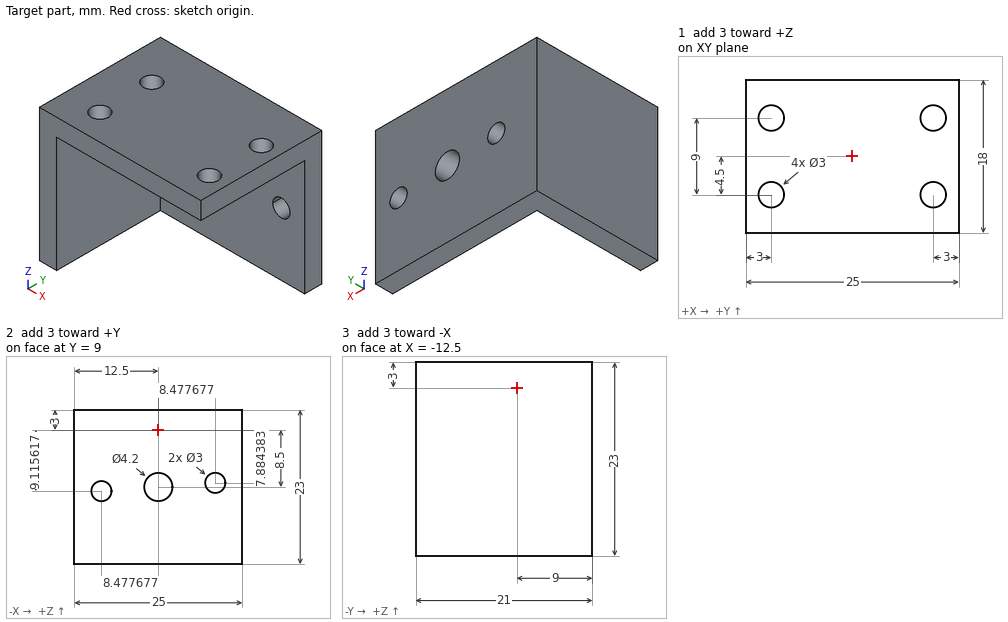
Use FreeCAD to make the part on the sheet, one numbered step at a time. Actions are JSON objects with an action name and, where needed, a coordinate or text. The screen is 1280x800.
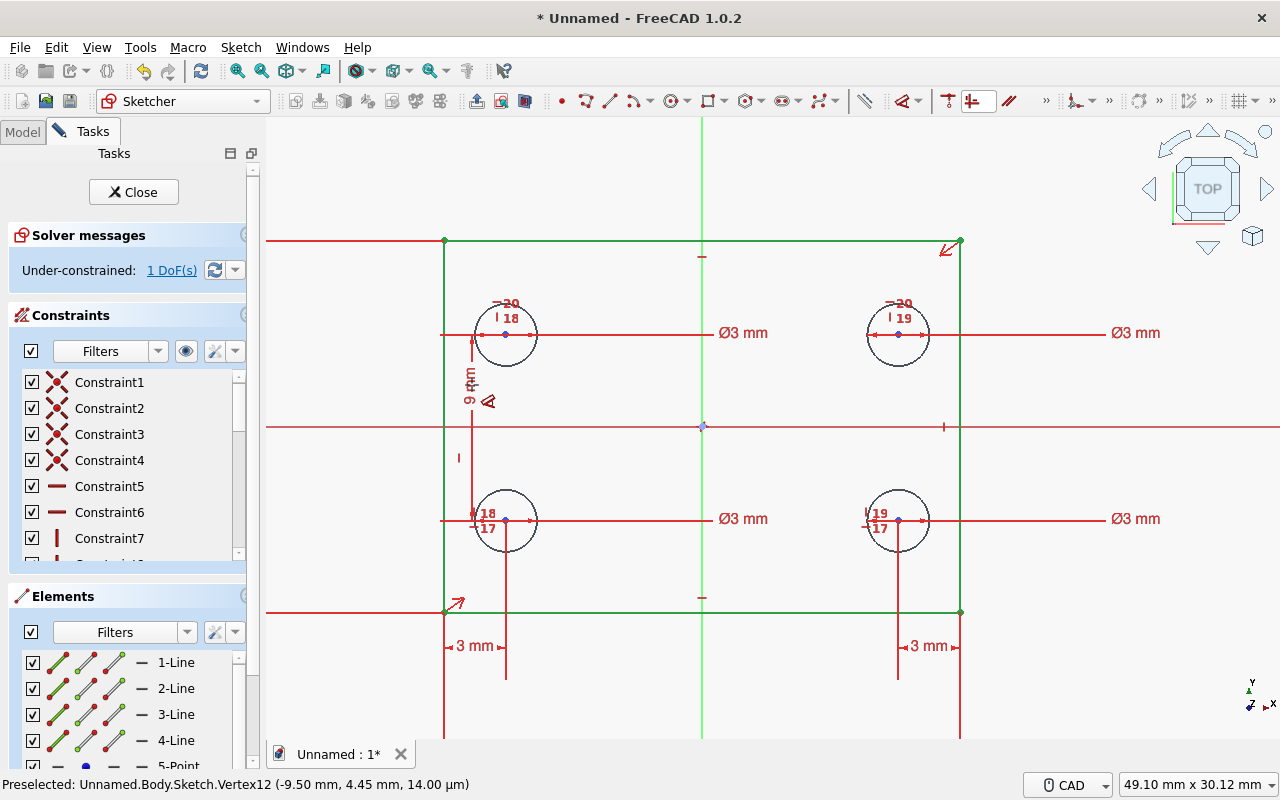
{"action": "left_click", "coordinate": [506, 521]}
{"action": "left_click", "coordinate": [472, 474]}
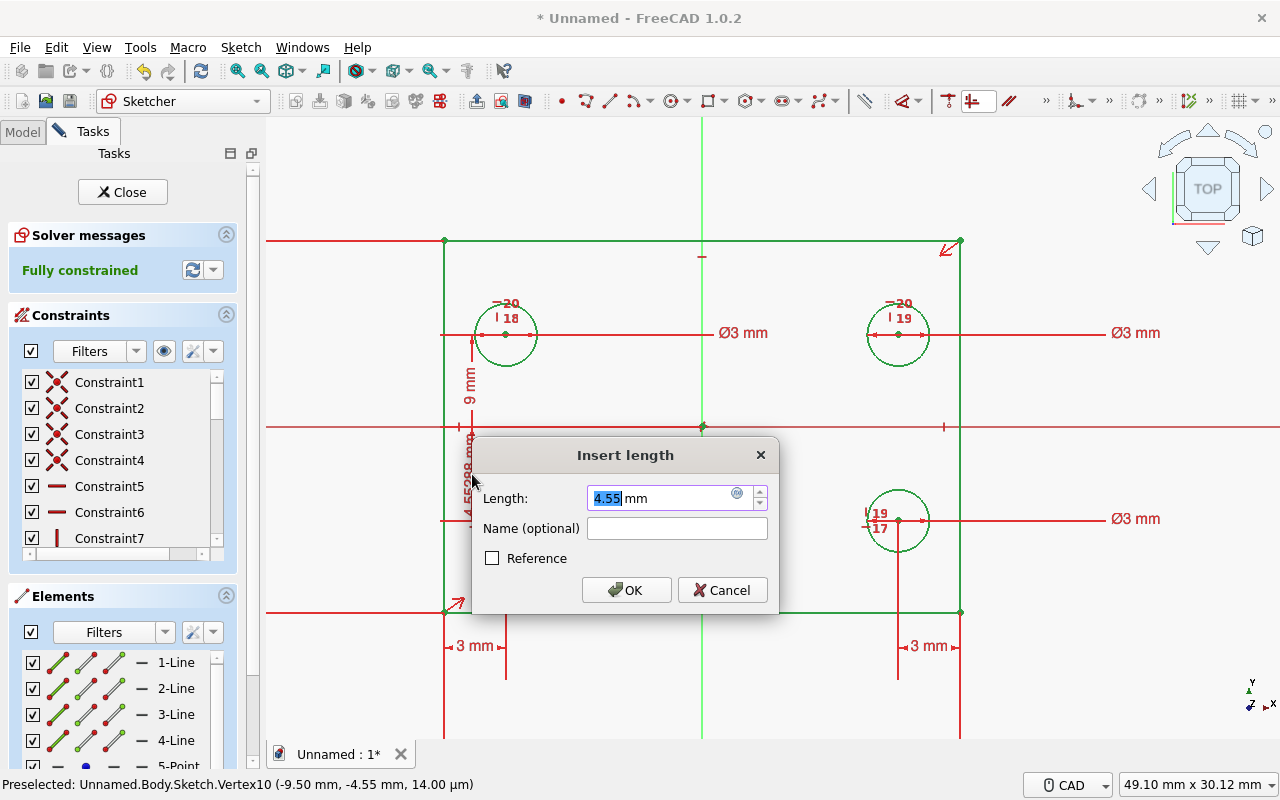
{"action": "type", "text": "4.5"}
{"action": "key", "text": "Return"}
{"action": "key", "text": "Escape"}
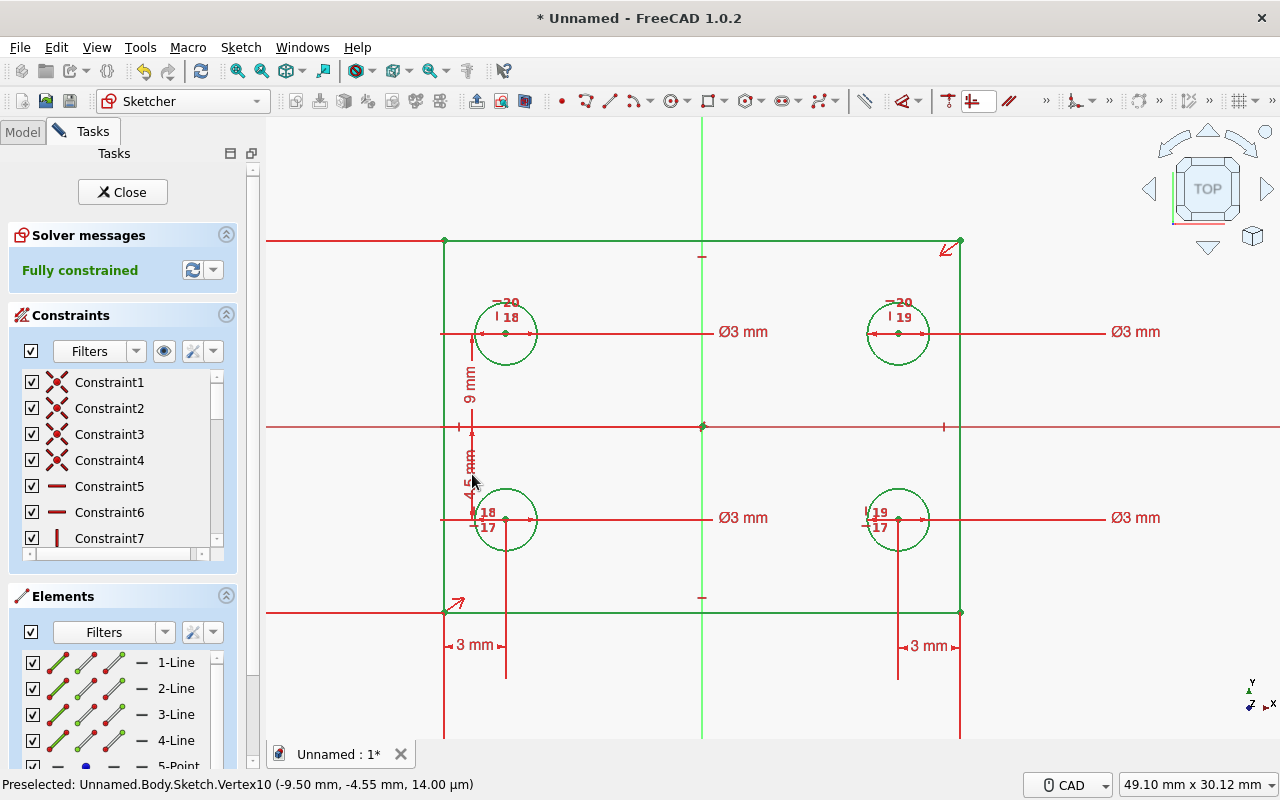
{"action": "left_click", "coordinate": [123, 192]}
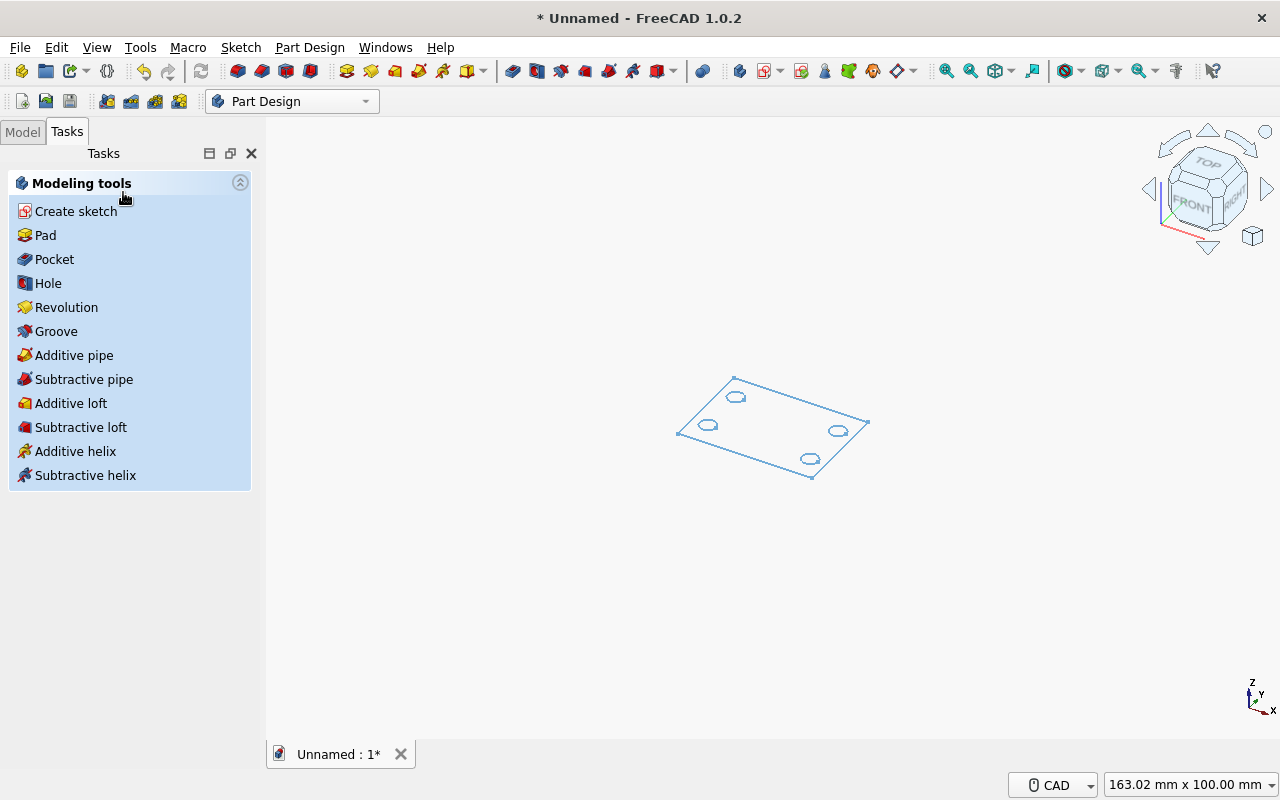
{"action": "left_click", "coordinate": [348, 72]}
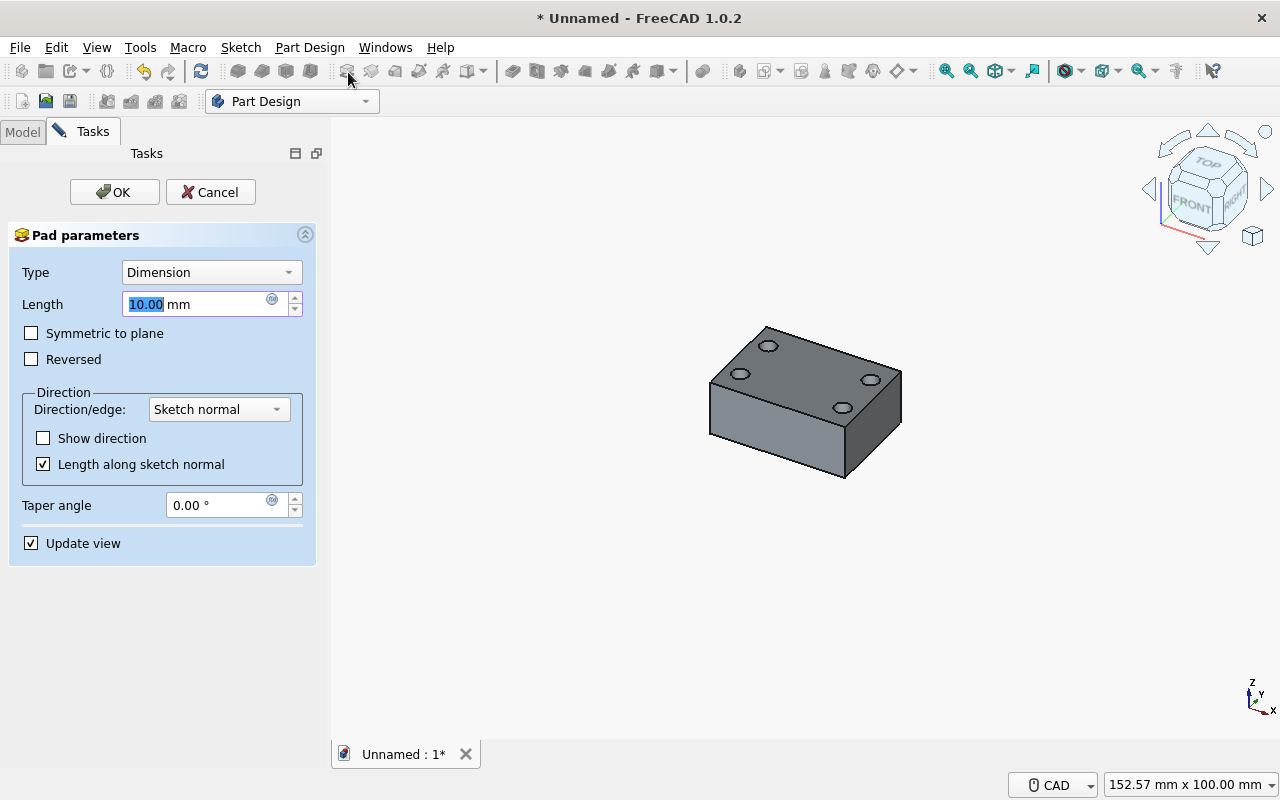
{"action": "type", "text": "3"}
{"action": "key", "text": "Tab"}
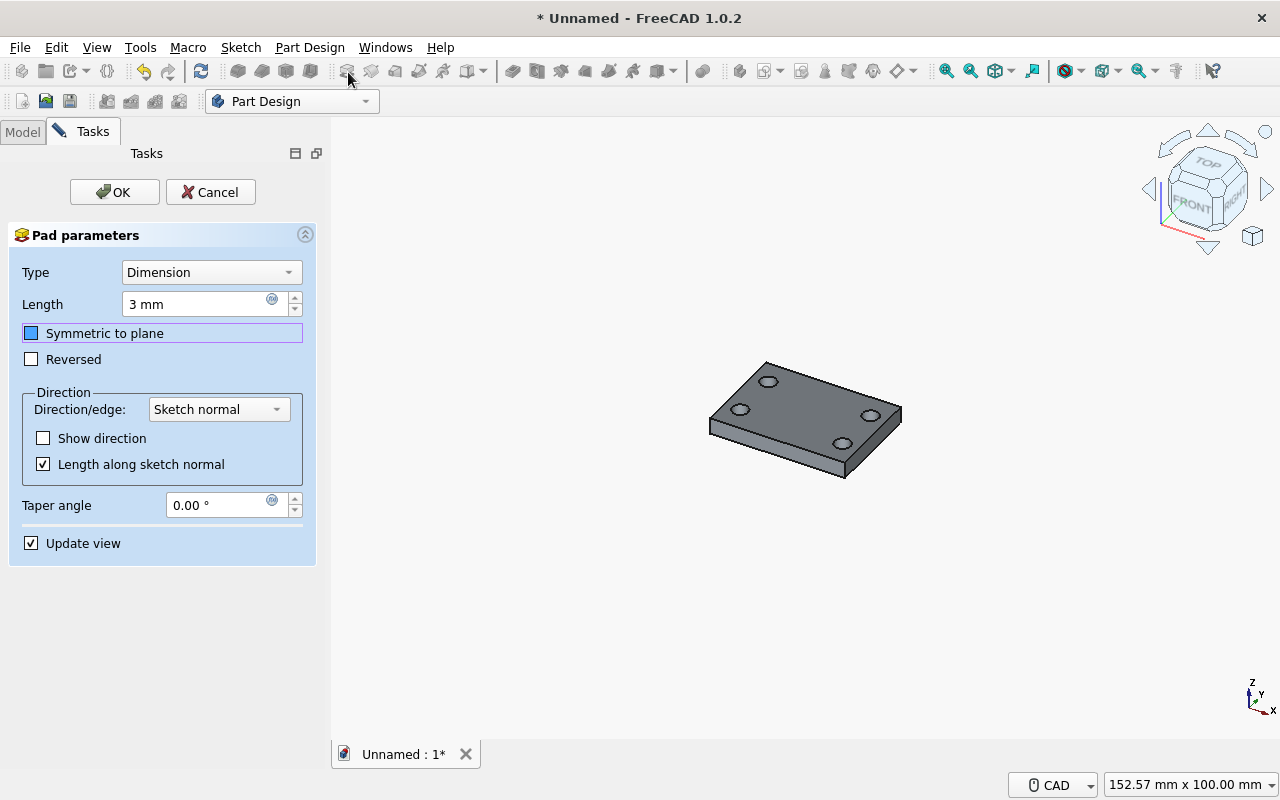
{"action": "left_click", "coordinate": [115, 192]}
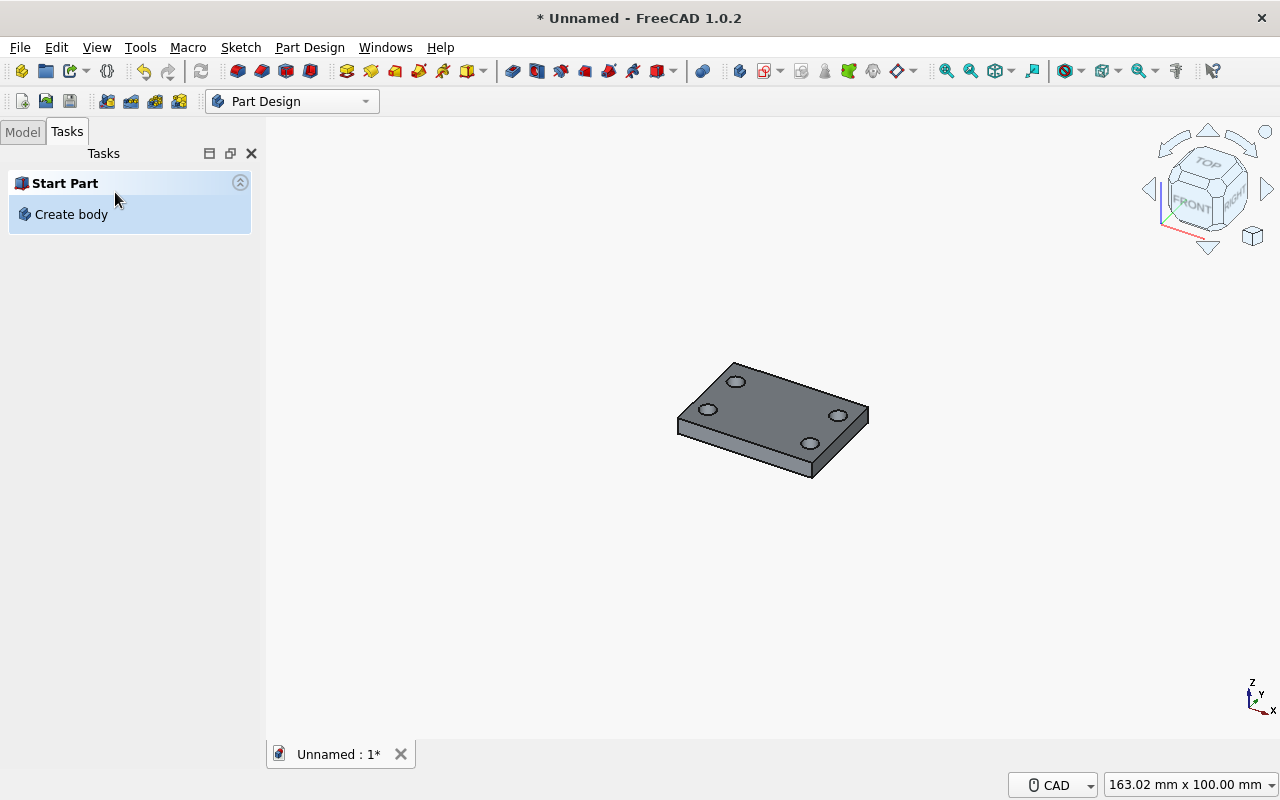
{"action": "left_click", "coordinate": [948, 72]}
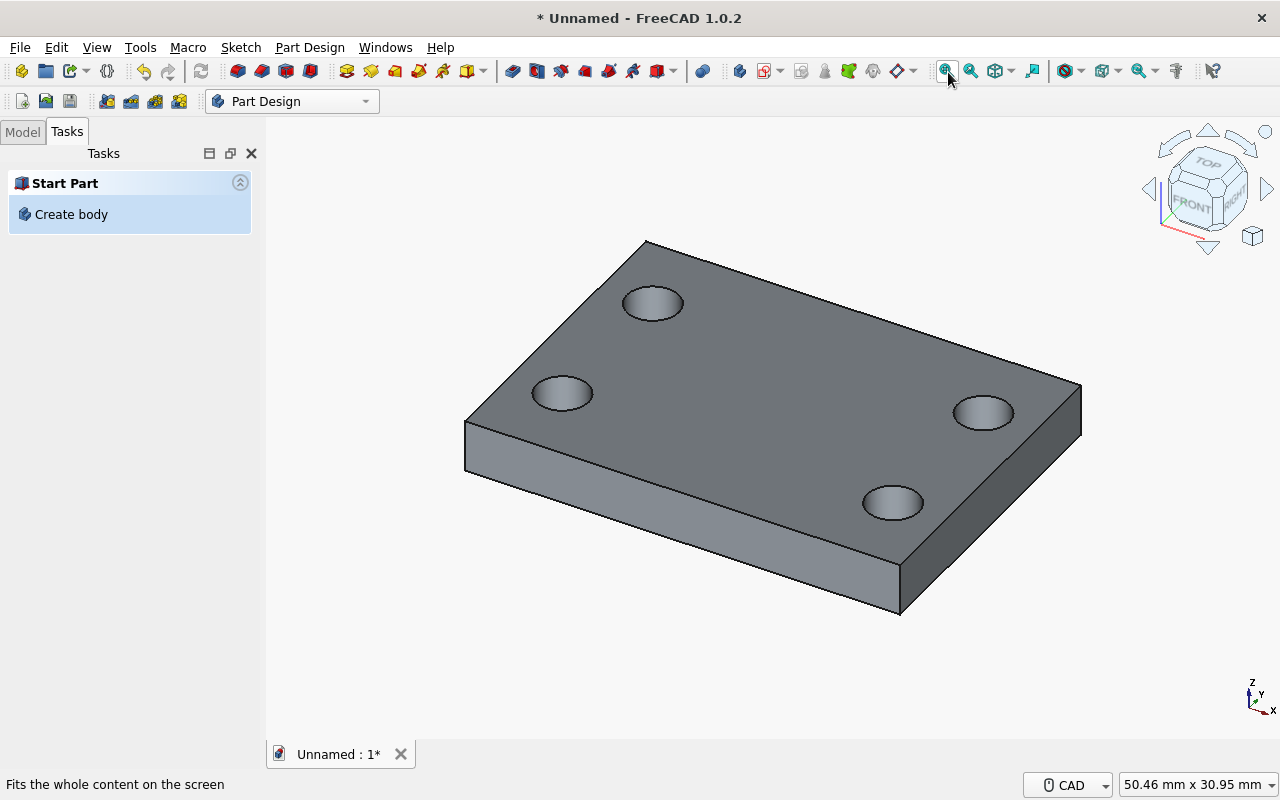
{"action": "key", "text": "4"}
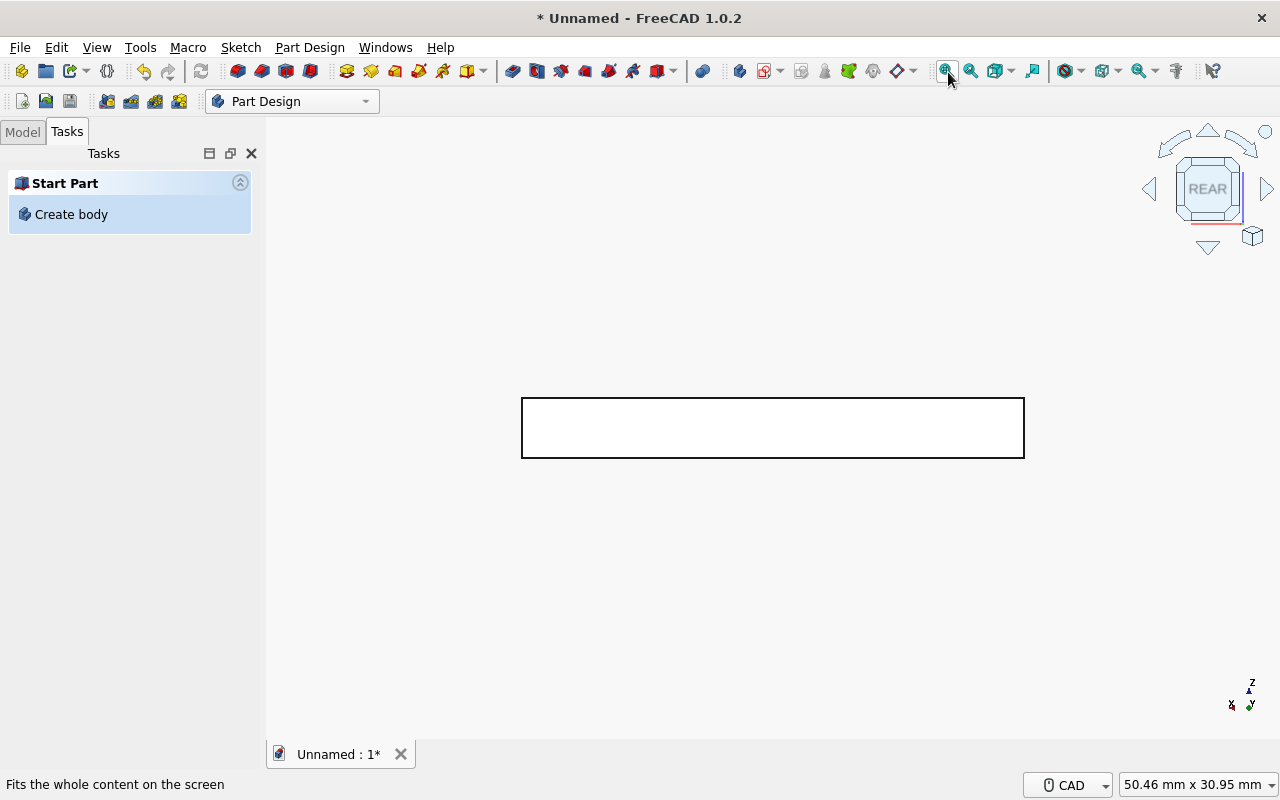
{"action": "left_click", "coordinate": [558, 427]}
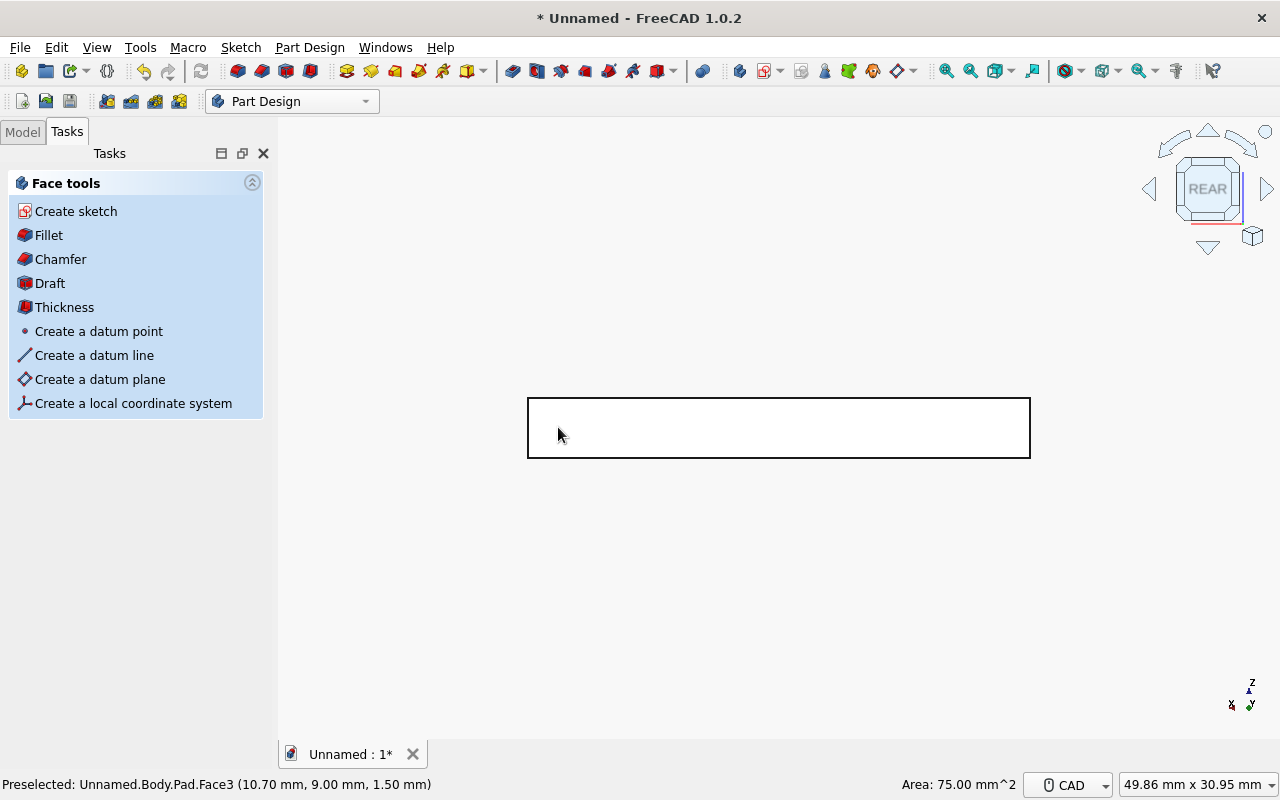
{"action": "left_click", "coordinate": [764, 72]}